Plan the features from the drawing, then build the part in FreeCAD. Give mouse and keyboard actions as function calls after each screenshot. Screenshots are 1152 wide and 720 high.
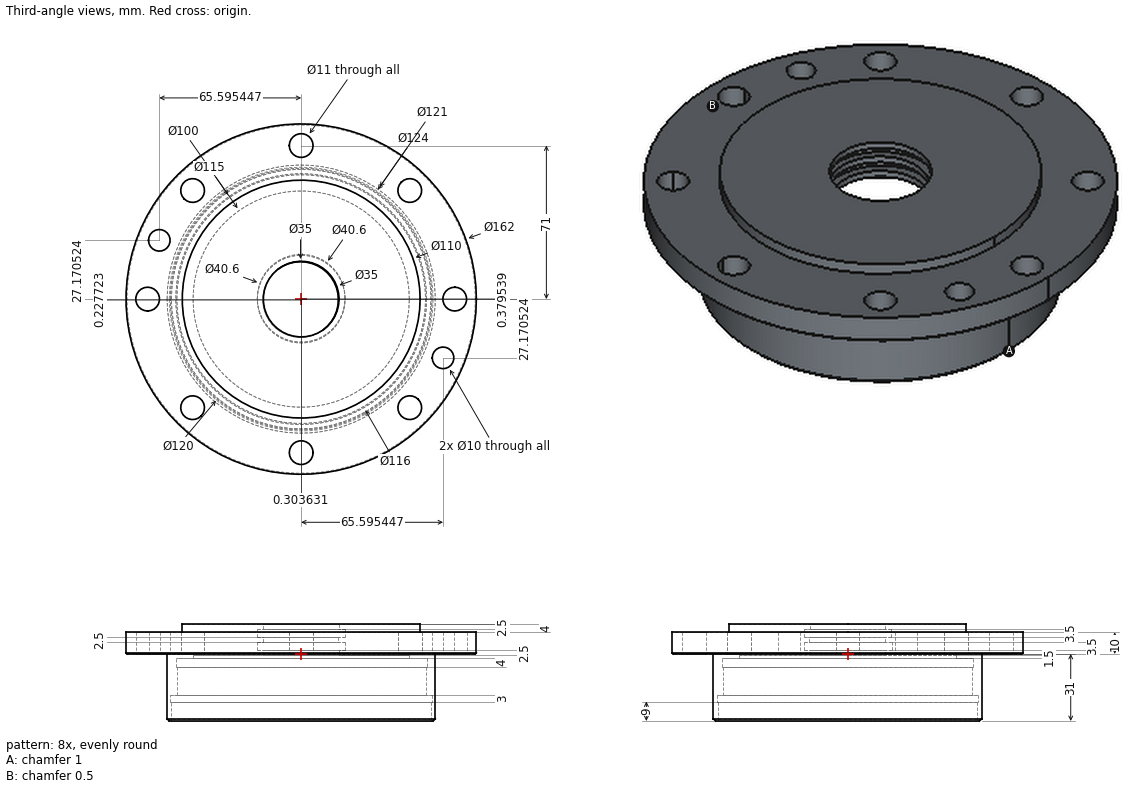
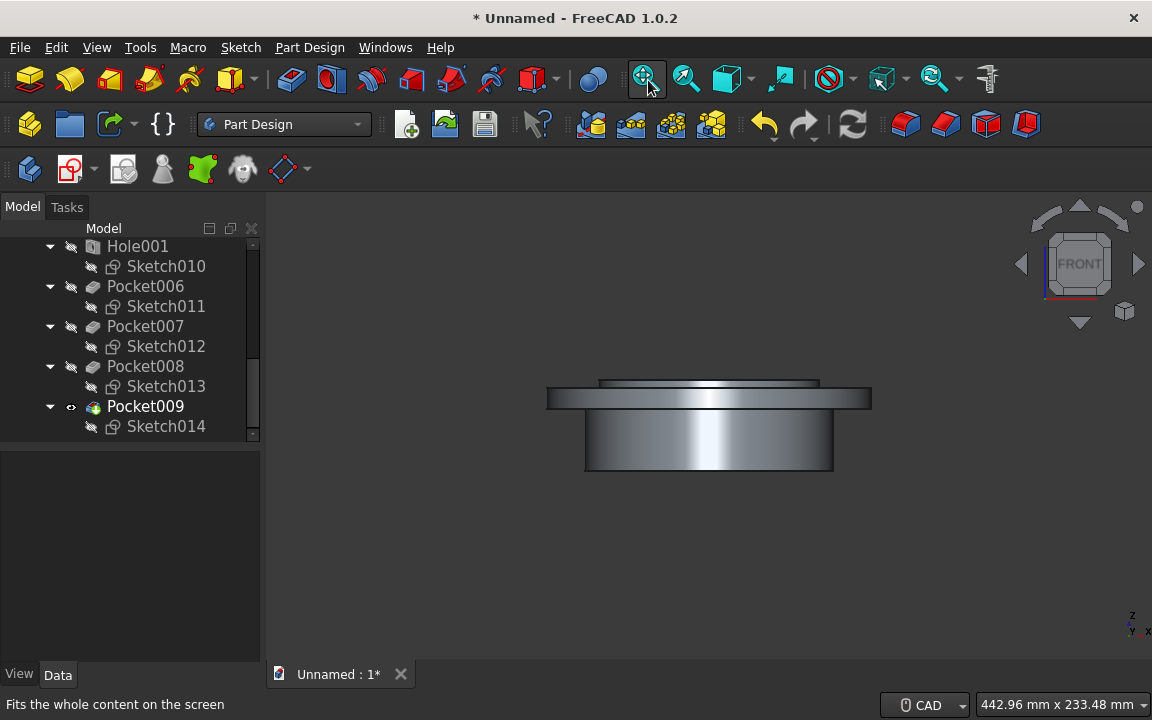
click(609, 470)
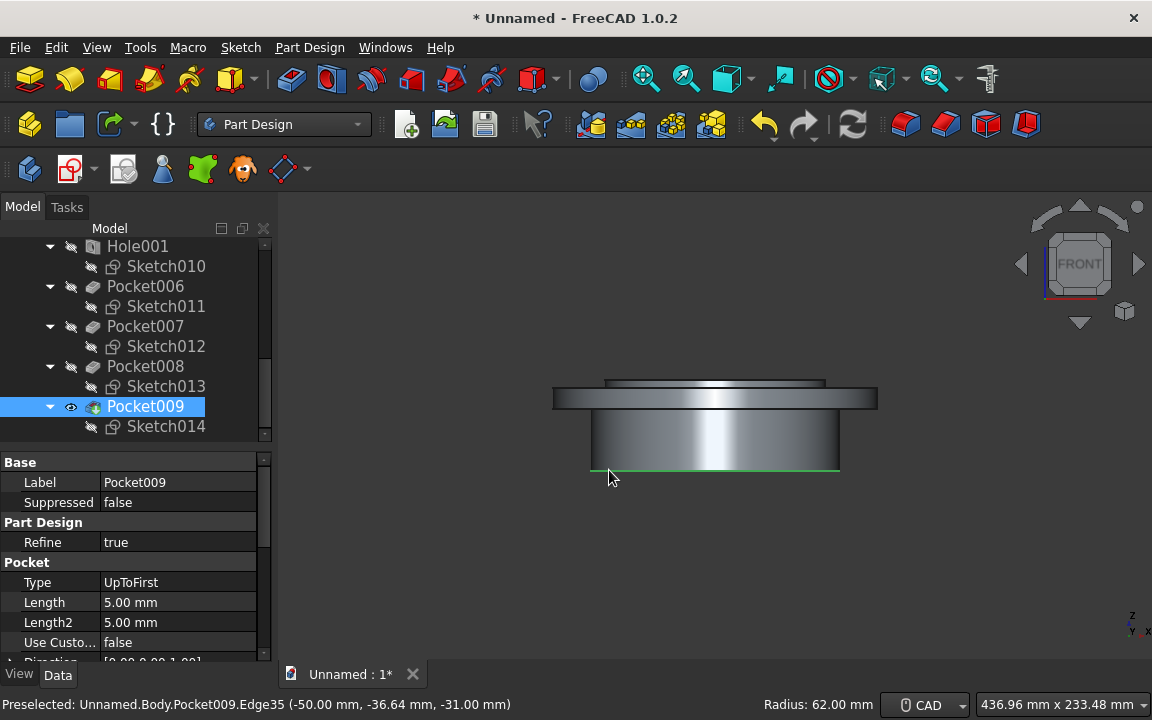
click(946, 124)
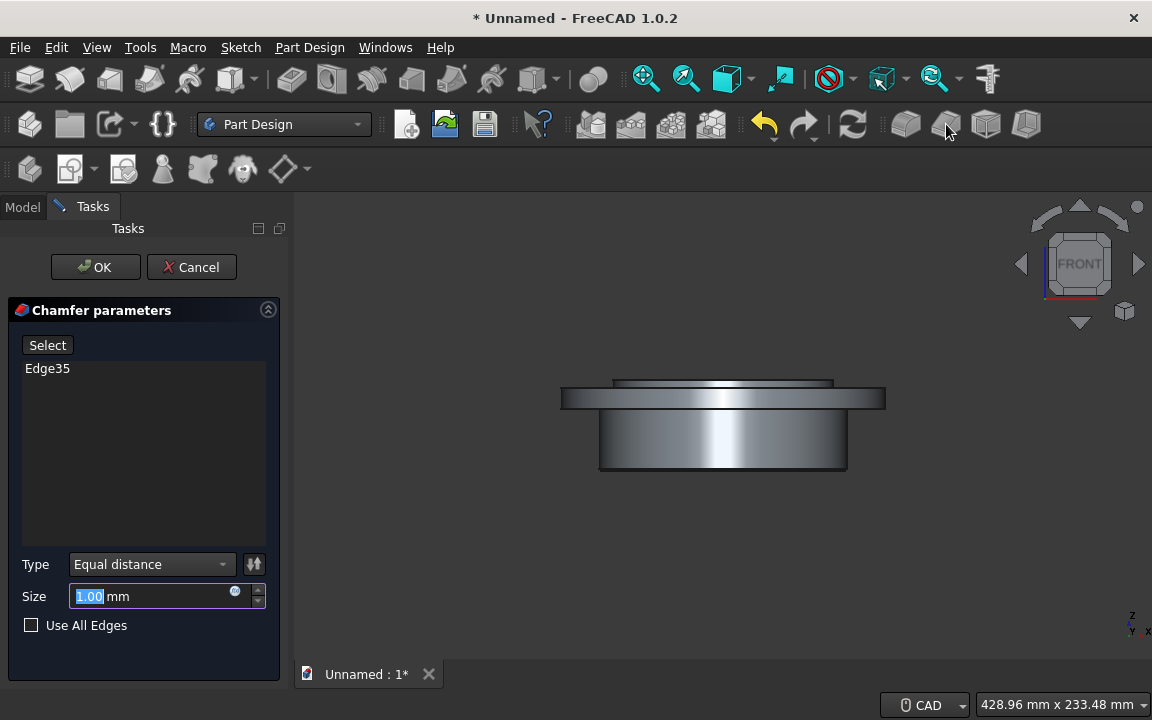
text(1)
key(Tab)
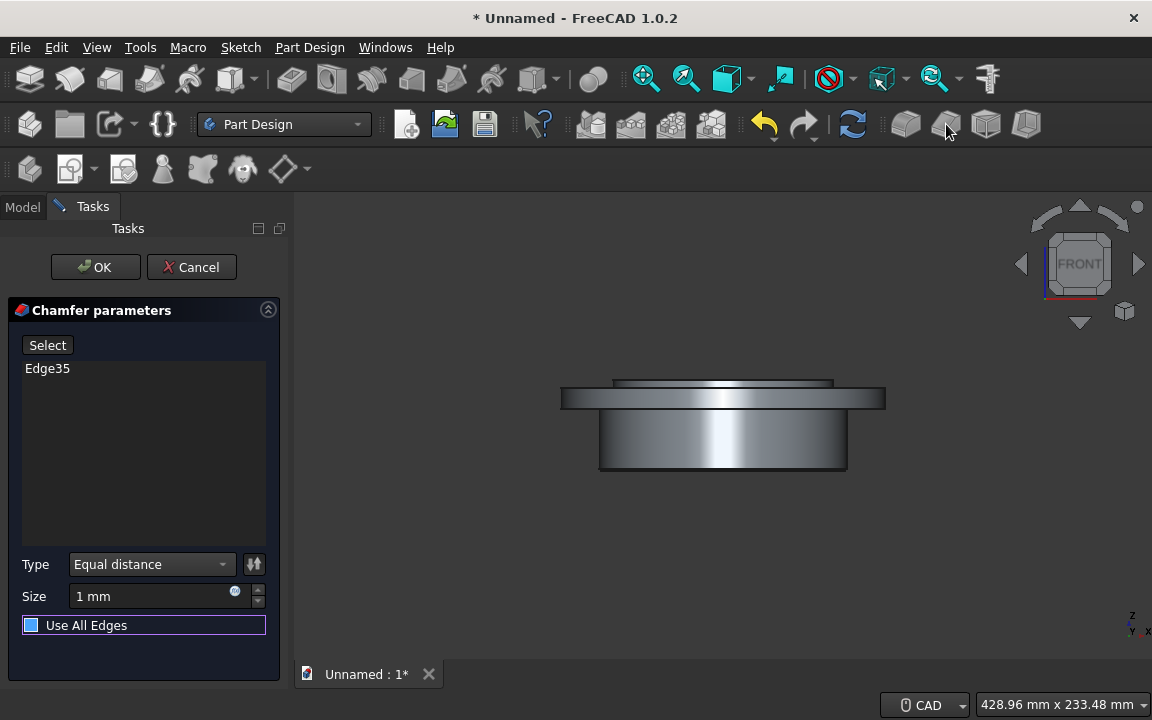
click(96, 267)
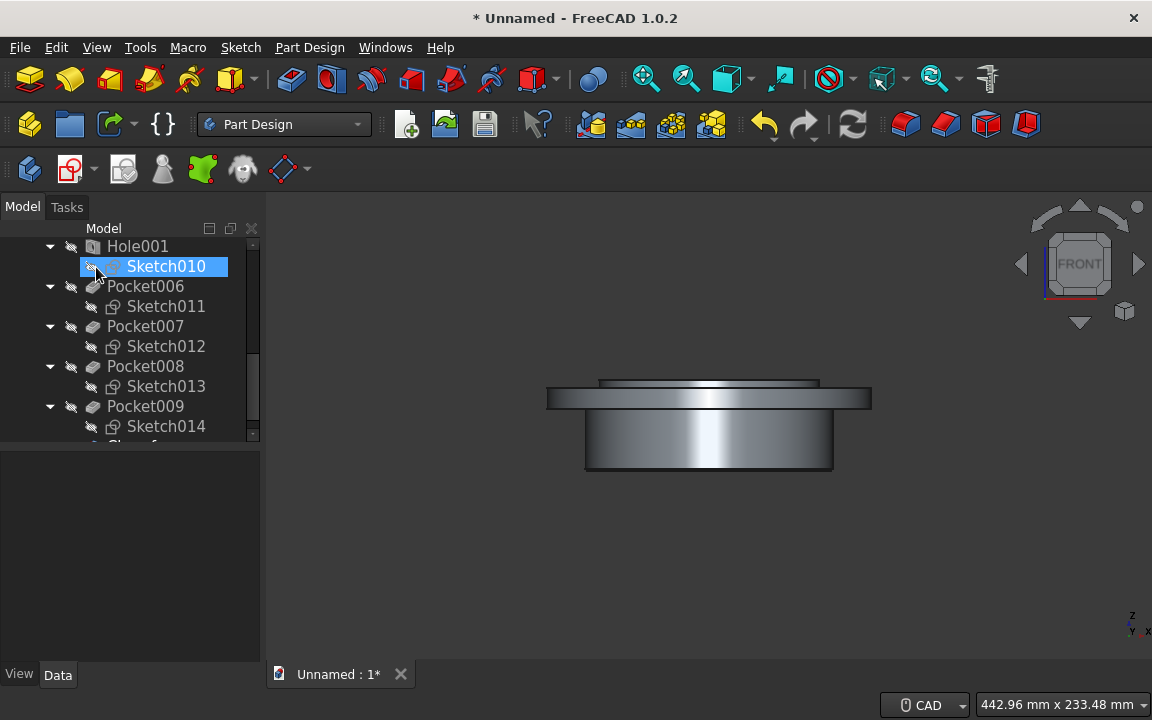
click(648, 80)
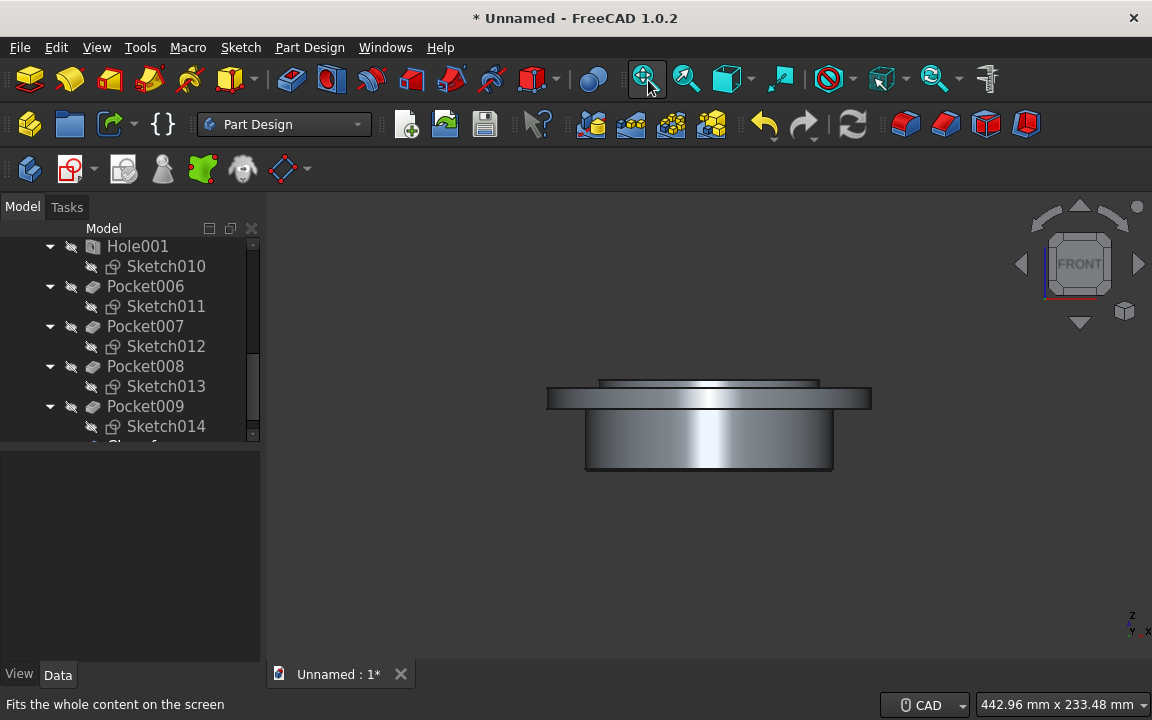
click(578, 407)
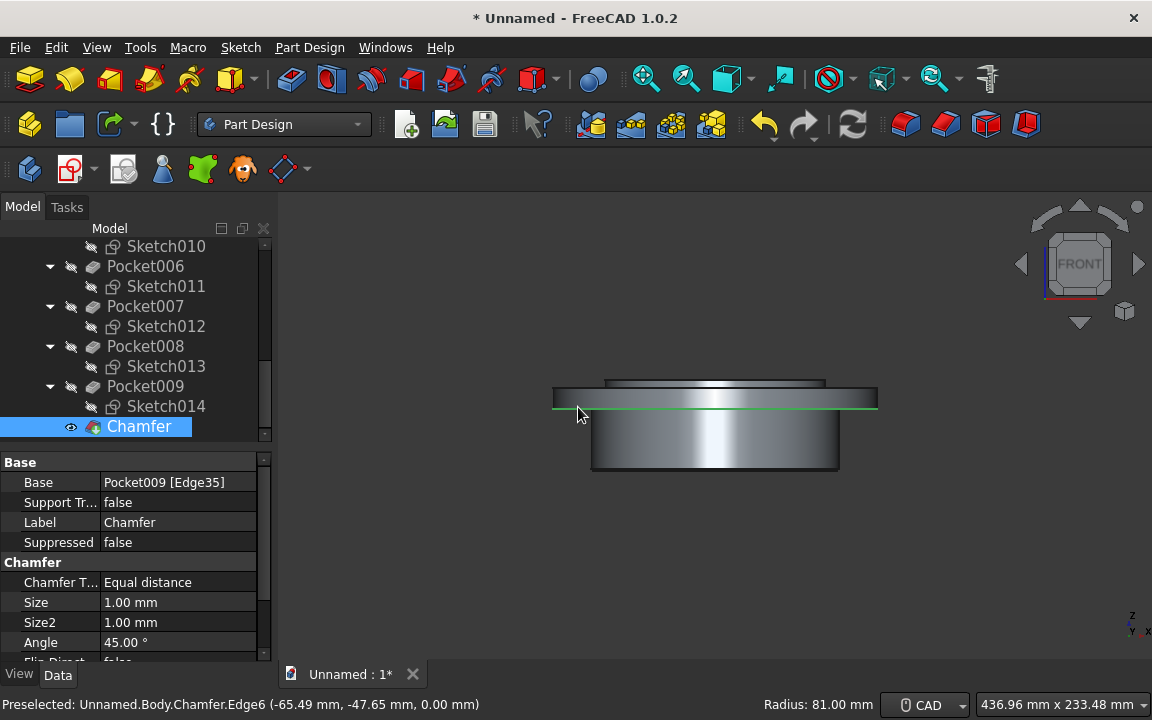
click(946, 124)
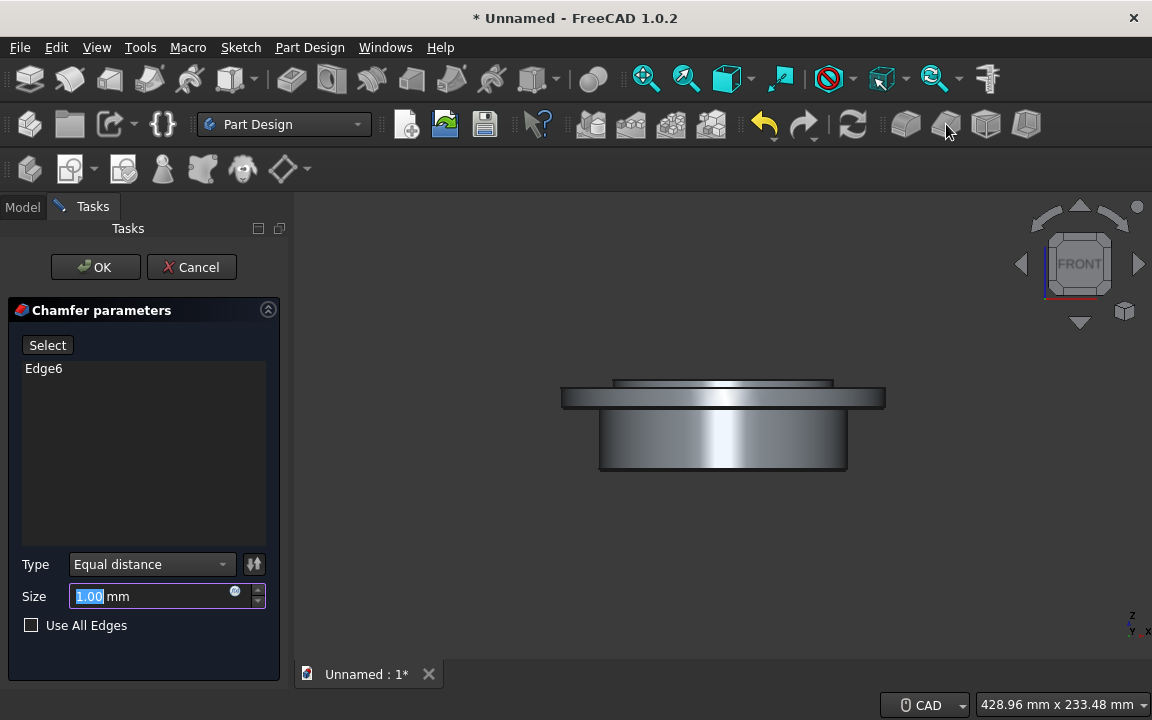
text(0.5)
key(Tab)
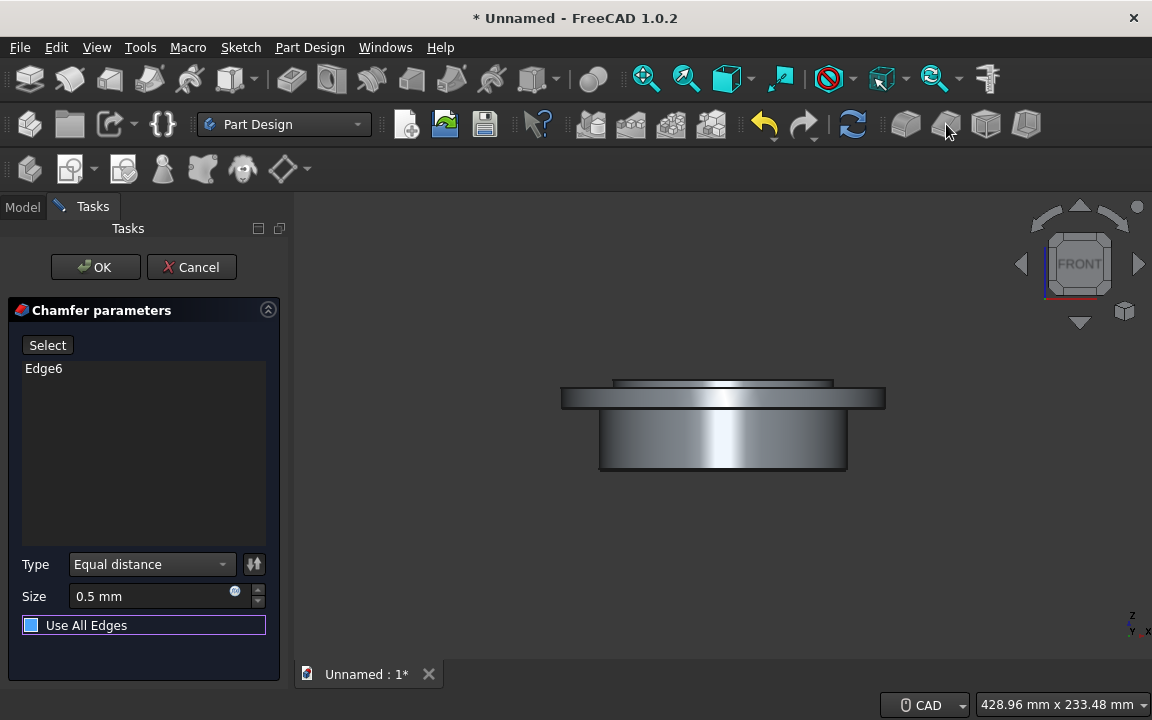
click(96, 267)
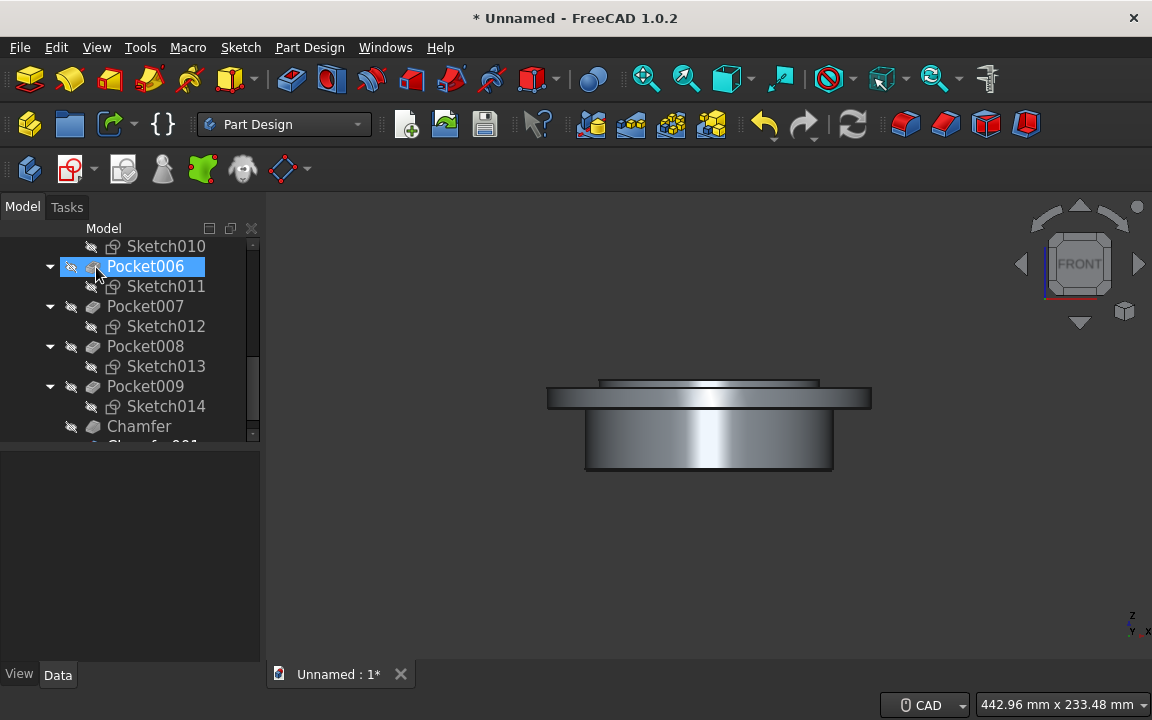
key(0)